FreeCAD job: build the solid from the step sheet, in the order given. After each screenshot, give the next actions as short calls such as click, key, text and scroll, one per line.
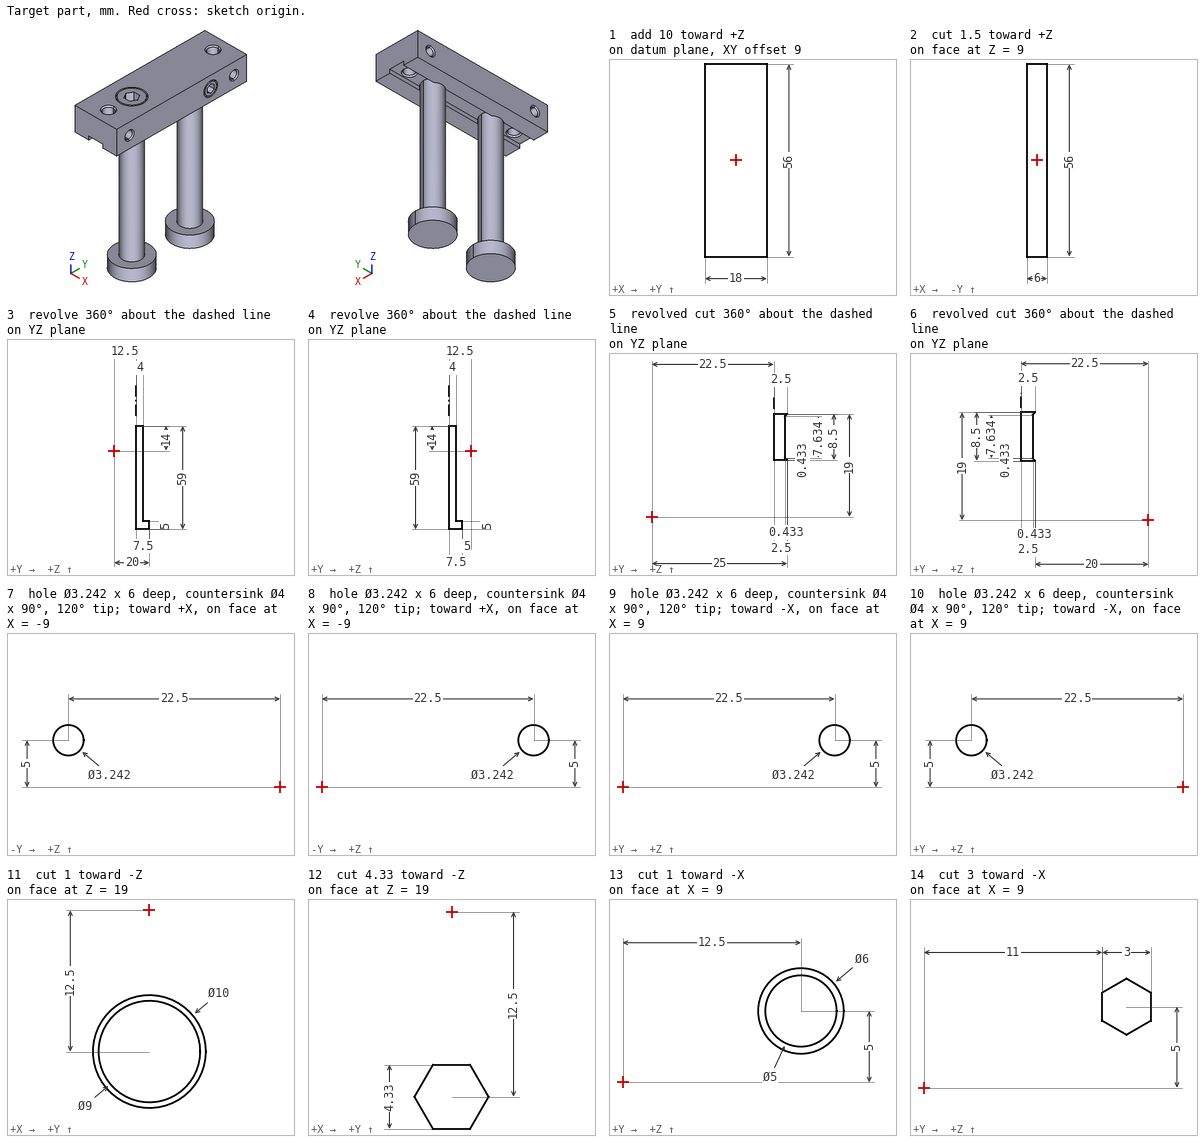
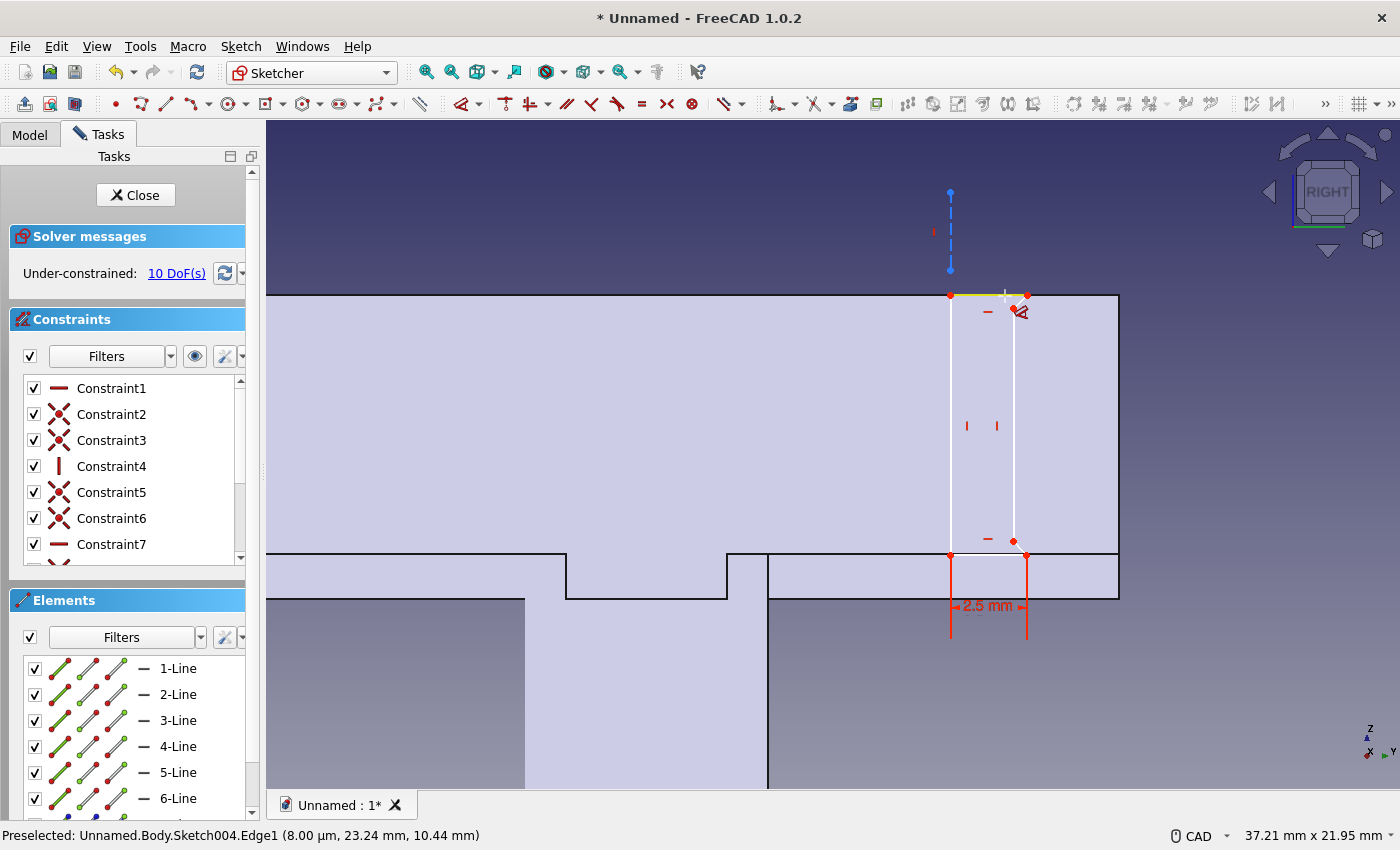
click(1004, 295)
click(989, 261)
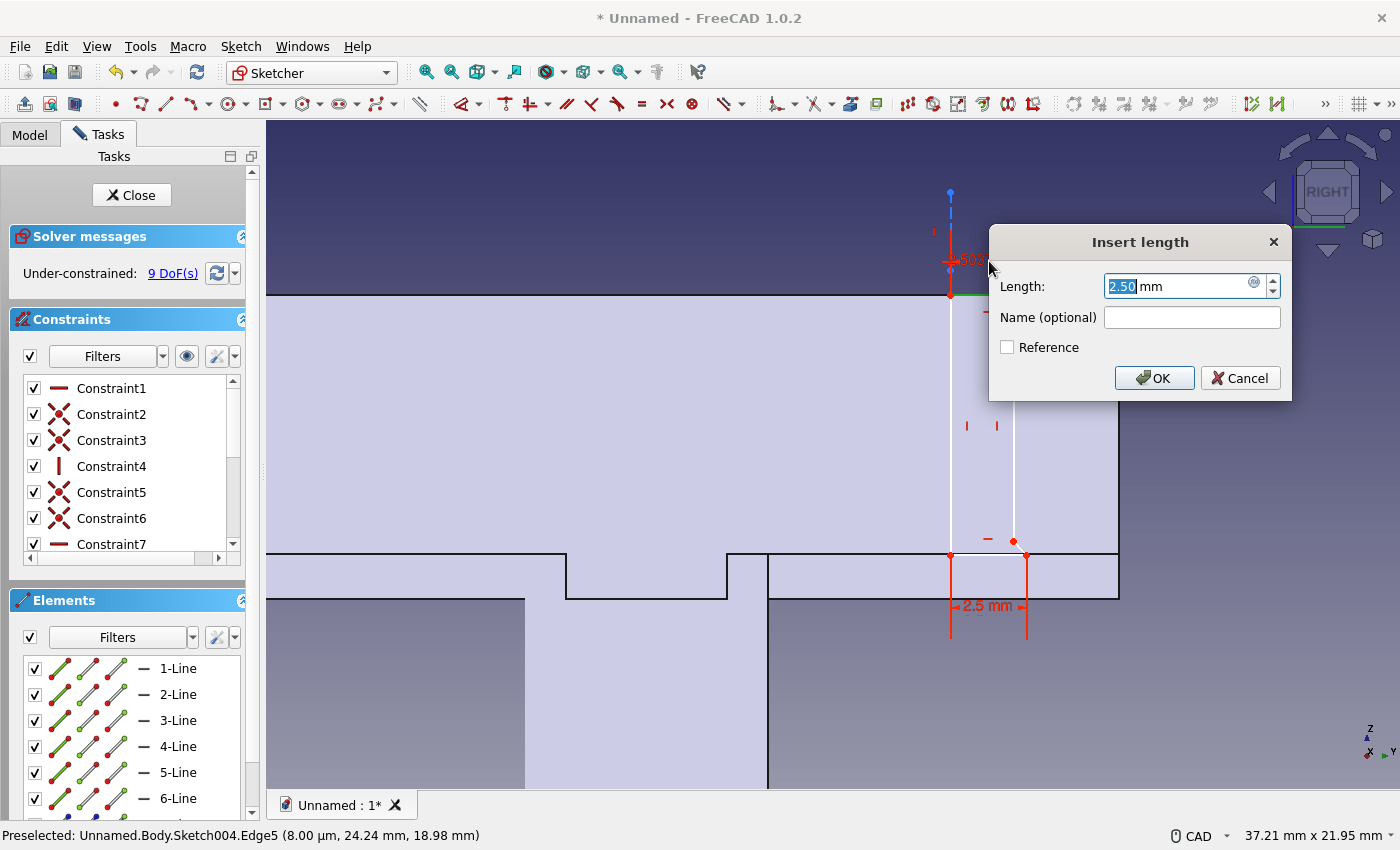
text(2.5)
key(Return)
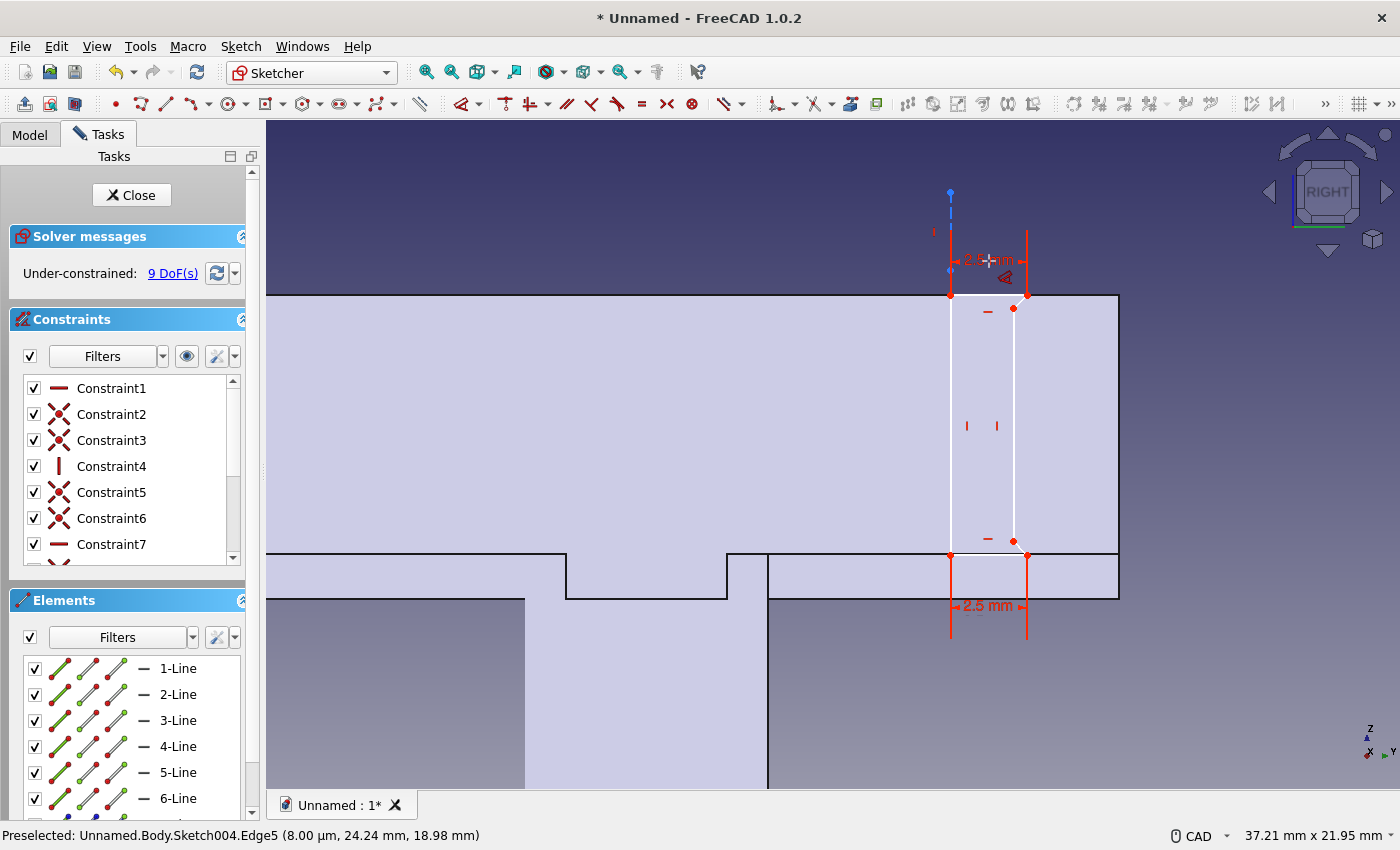
click(951, 373)
click(985, 425)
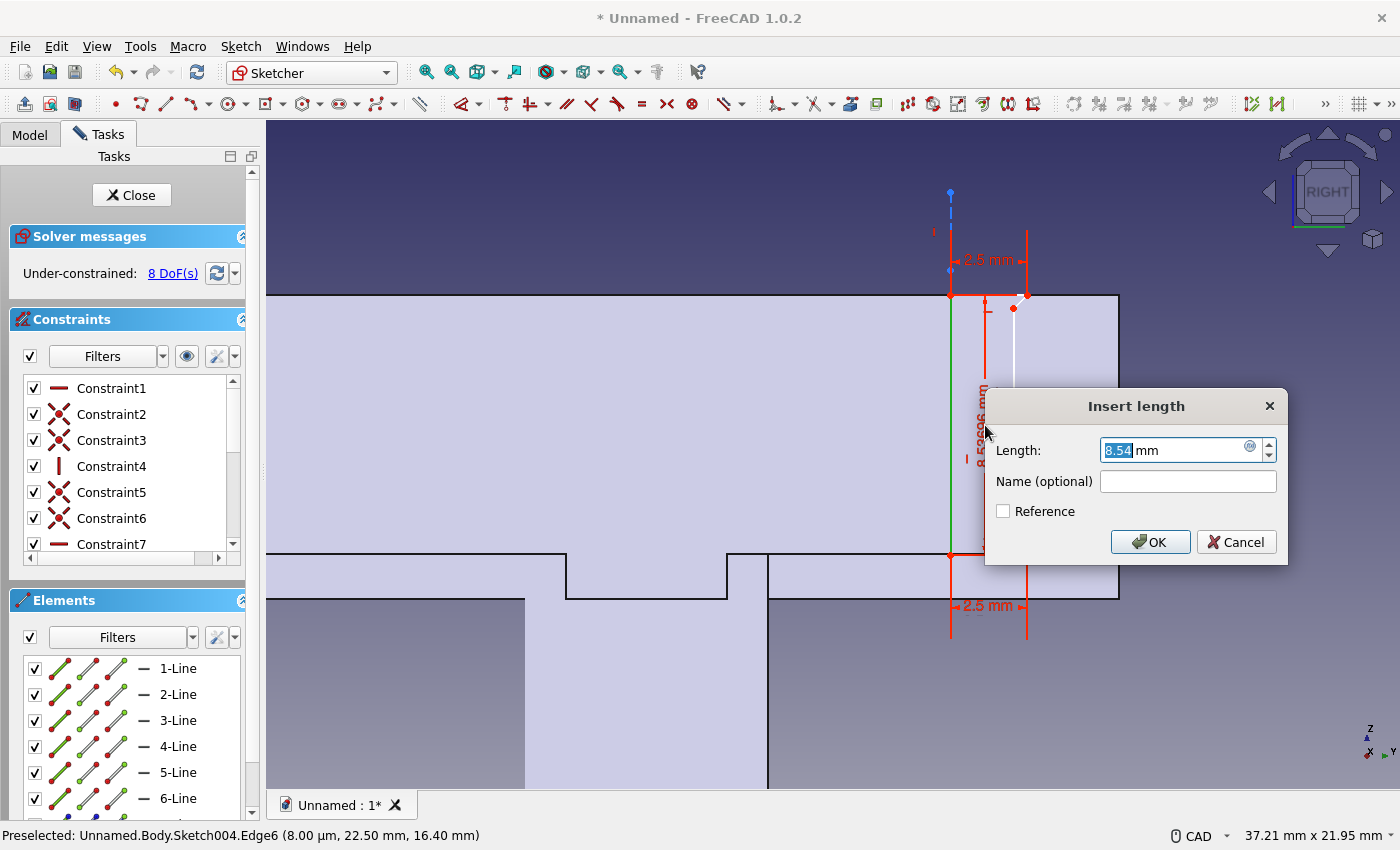
text(8.5)
key(Return)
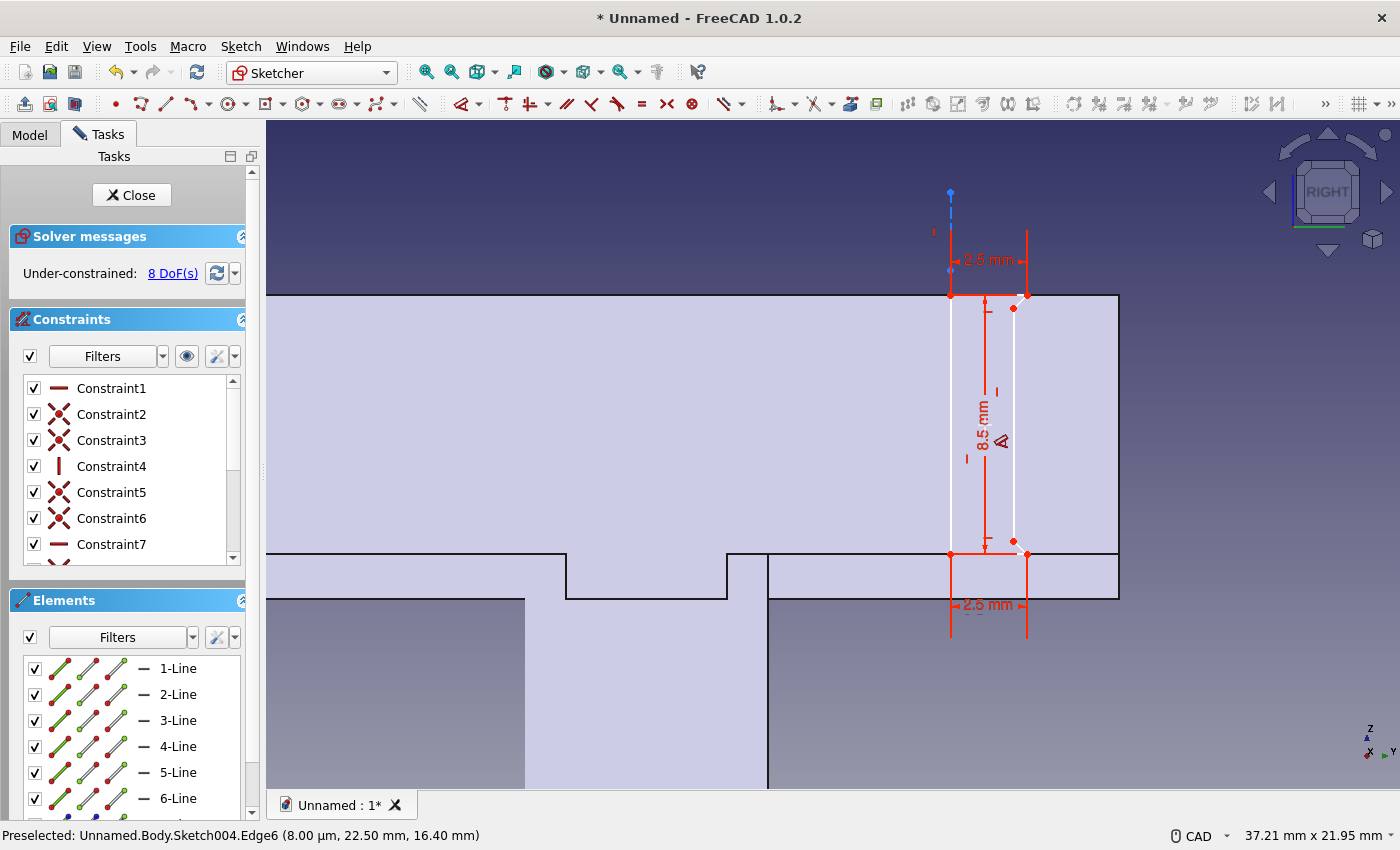
click(1027, 554)
click(661, 520)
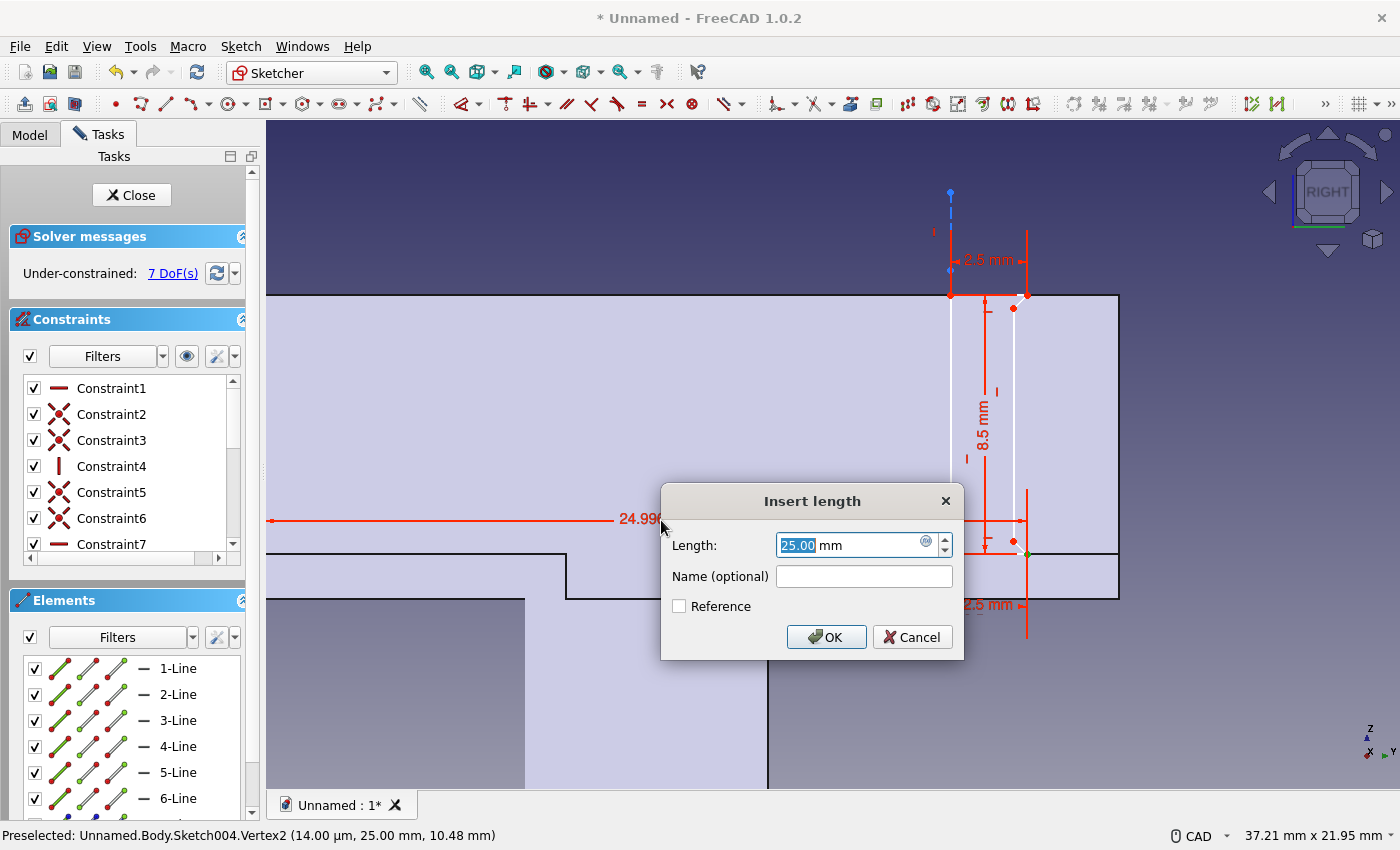
text(25)
key(Return)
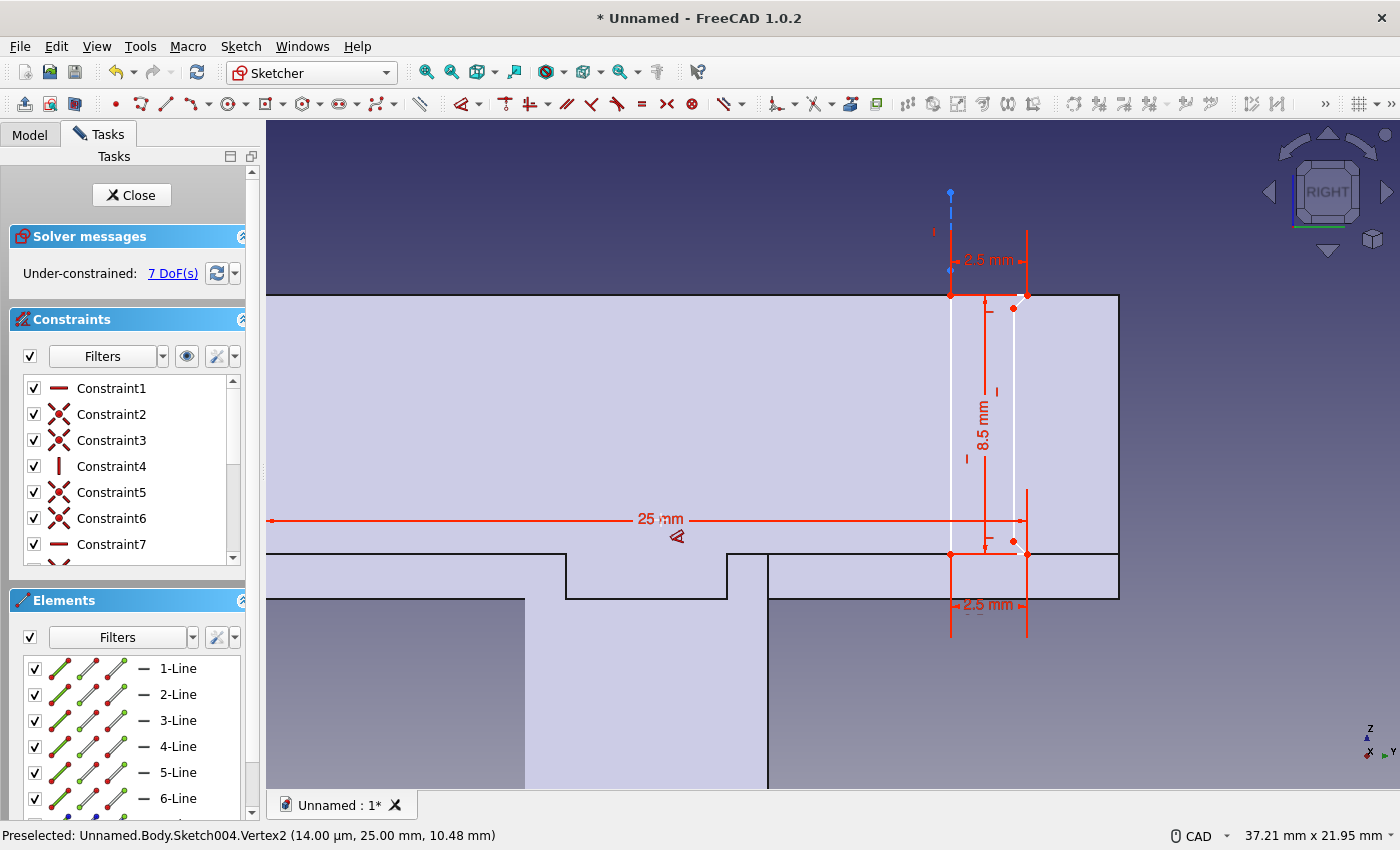
click(1027, 295)
click(1061, 528)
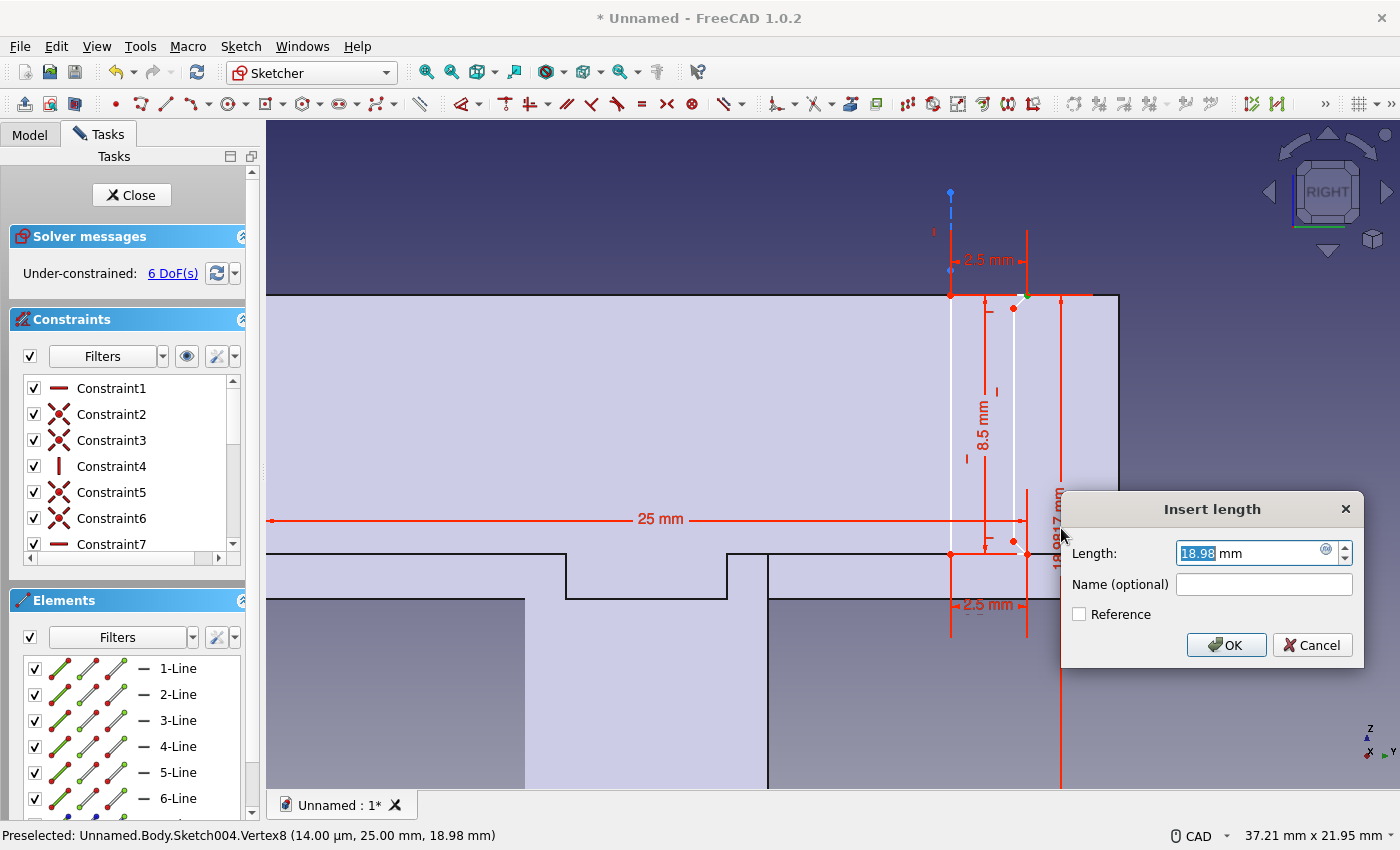
text(19)
key(Return)